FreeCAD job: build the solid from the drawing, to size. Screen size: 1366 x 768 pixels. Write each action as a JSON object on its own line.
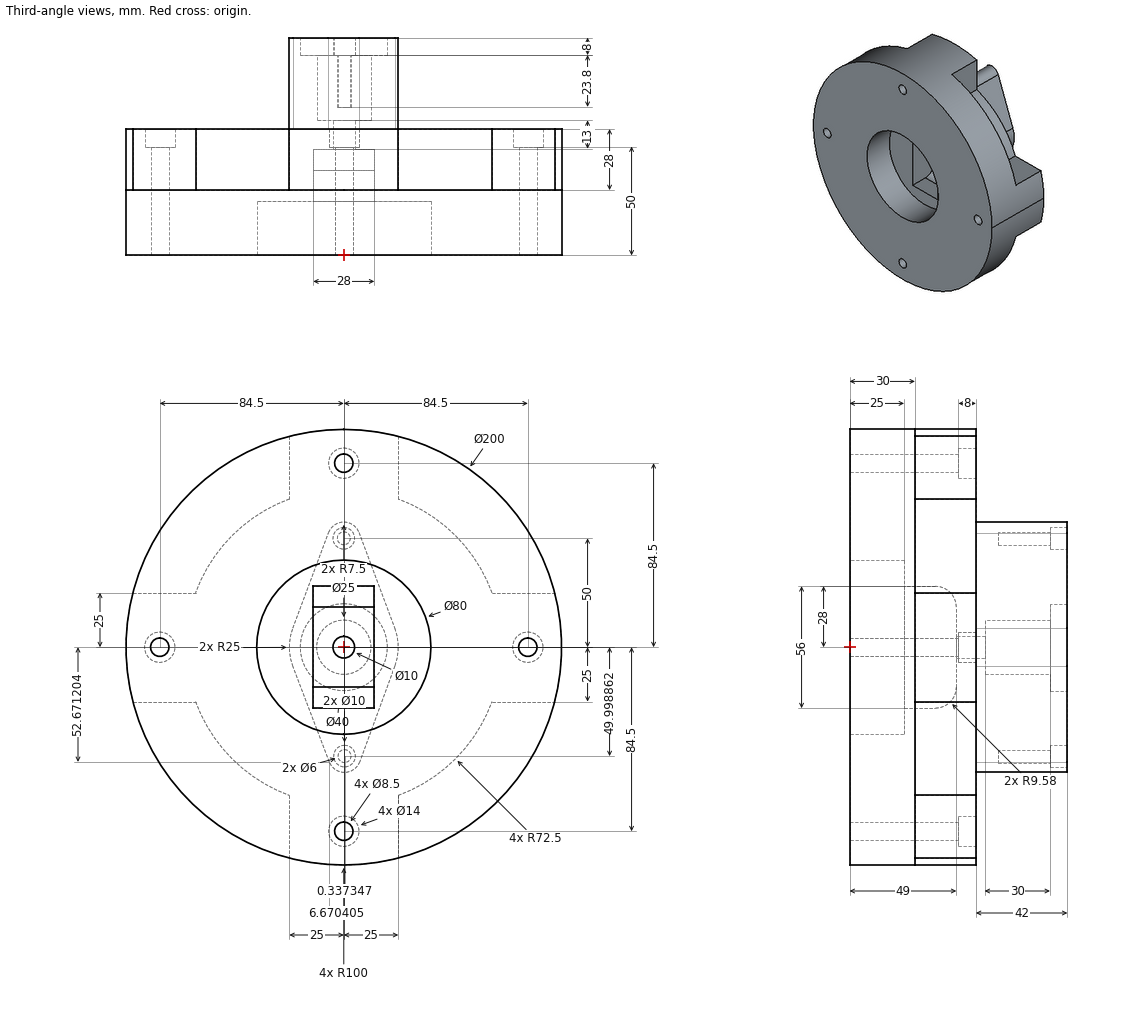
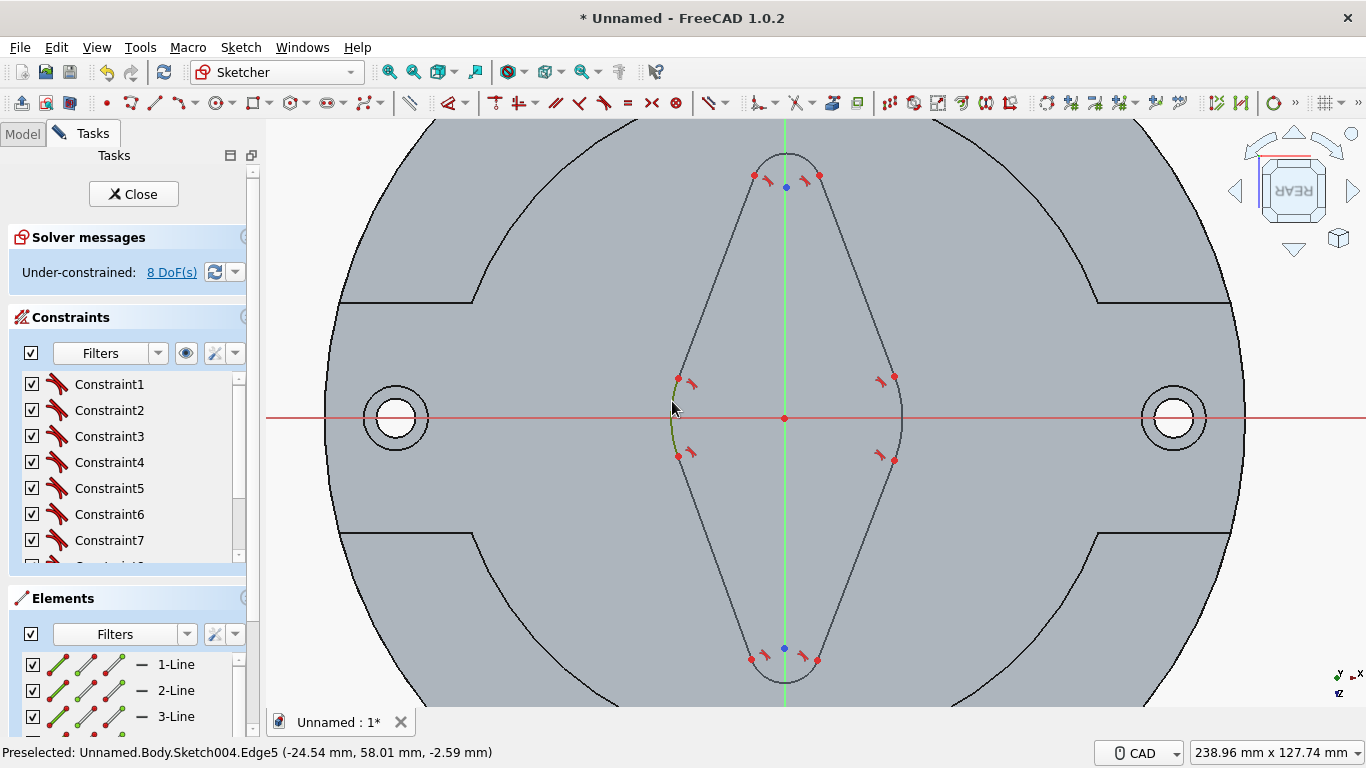
{"action": "left_click", "coordinate": [901, 436]}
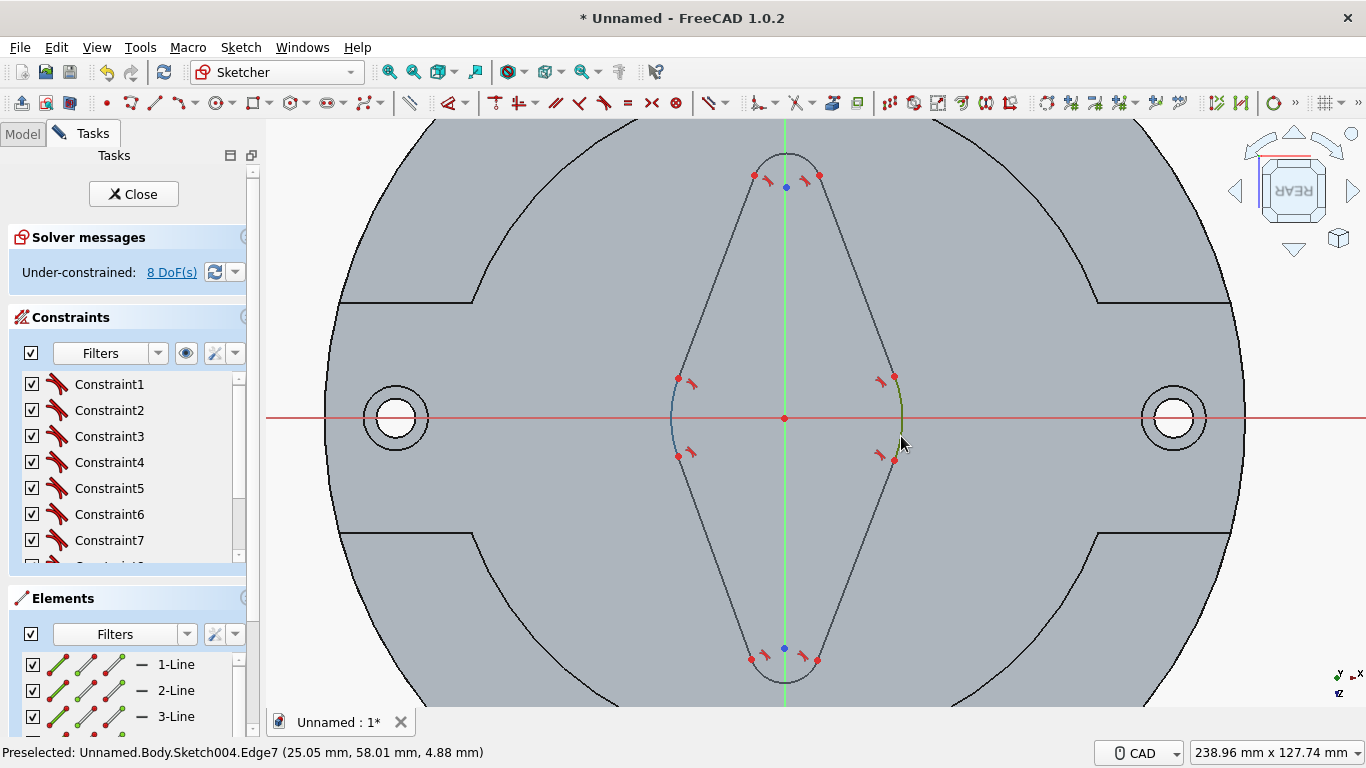
{"action": "key", "text": "e"}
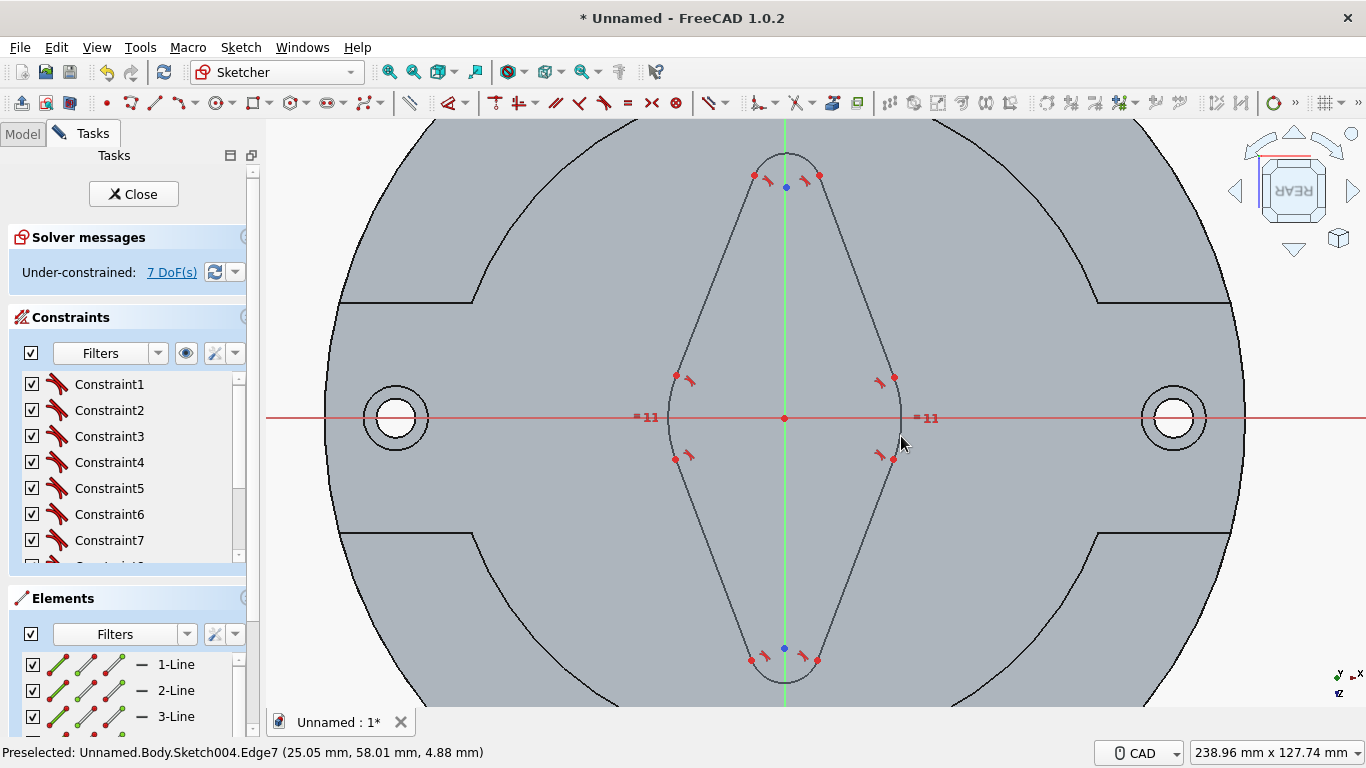
{"action": "left_click", "coordinate": [761, 674]}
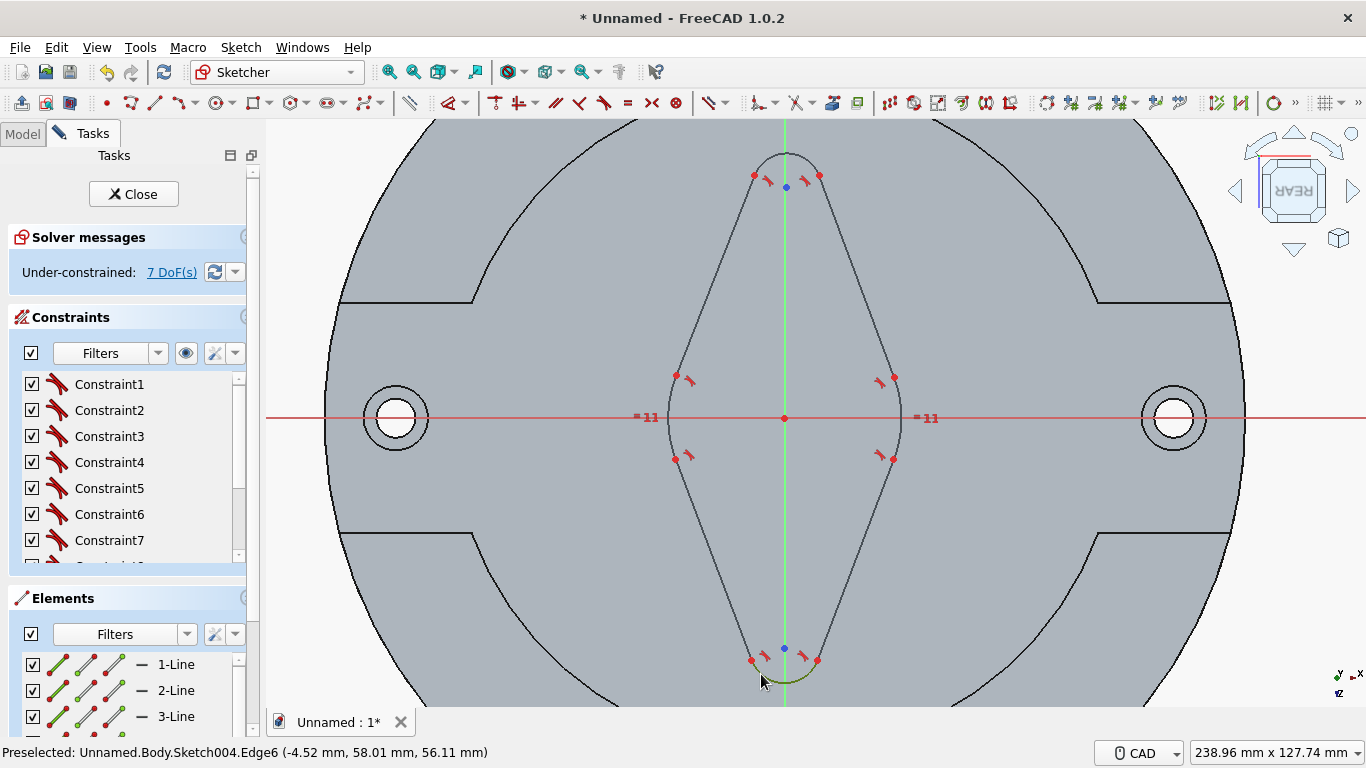
{"action": "left_click", "coordinate": [803, 157]}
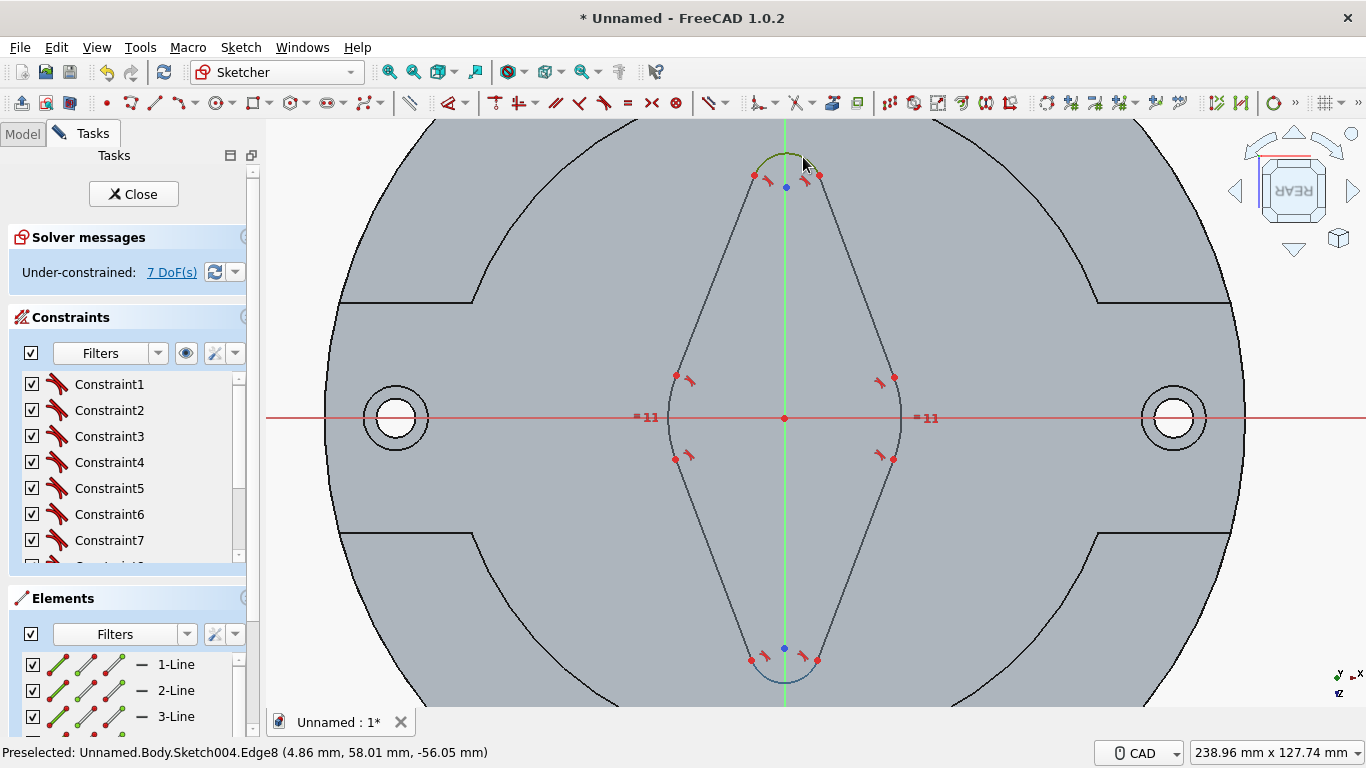
{"action": "key", "text": "e"}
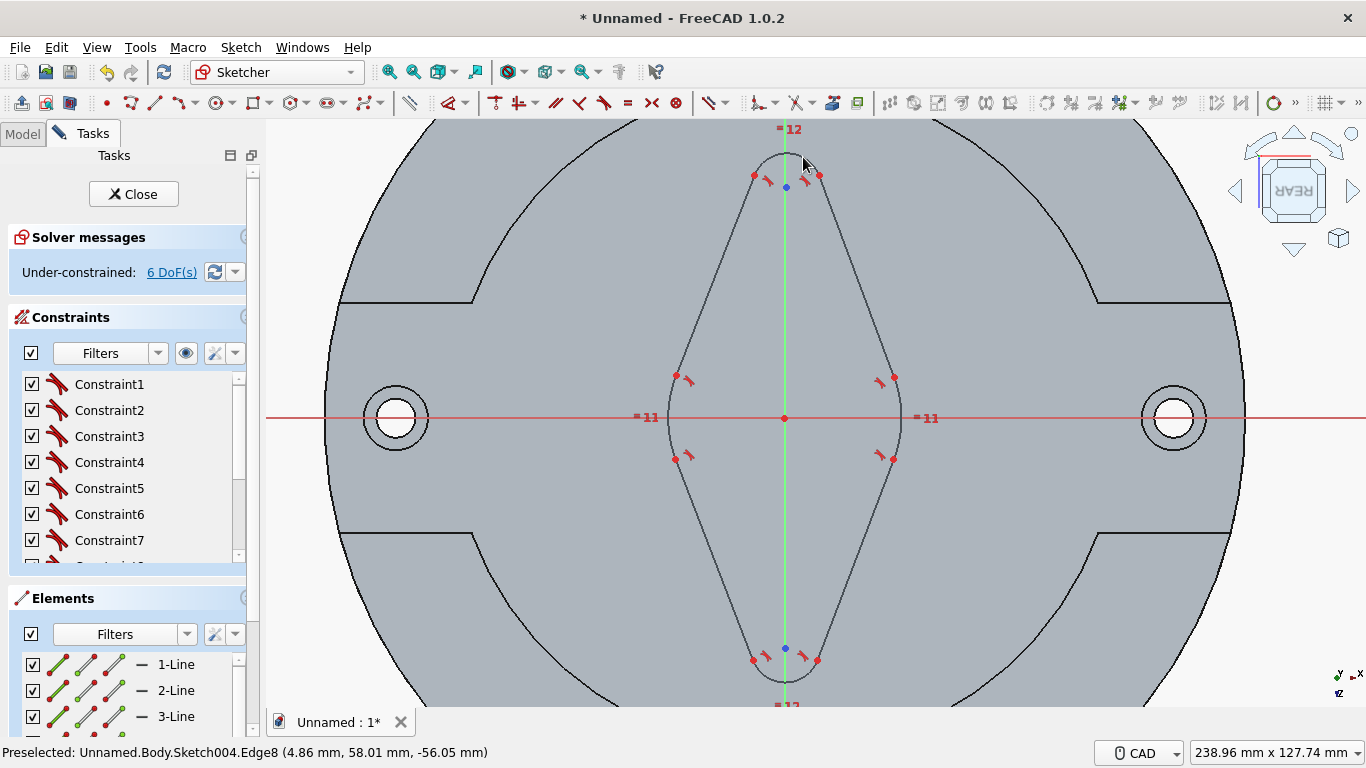
{"action": "left_click", "coordinate": [785, 648]}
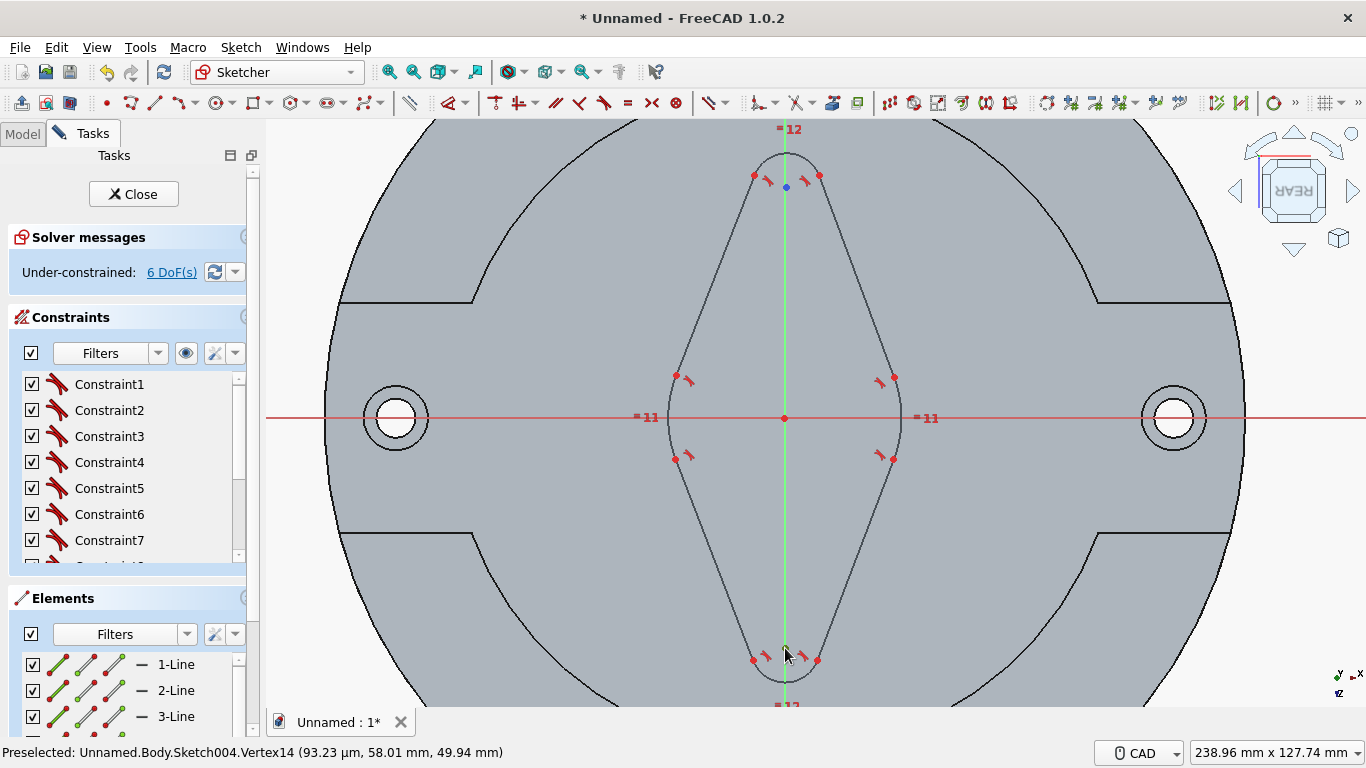
{"action": "left_click", "coordinate": [785, 641]}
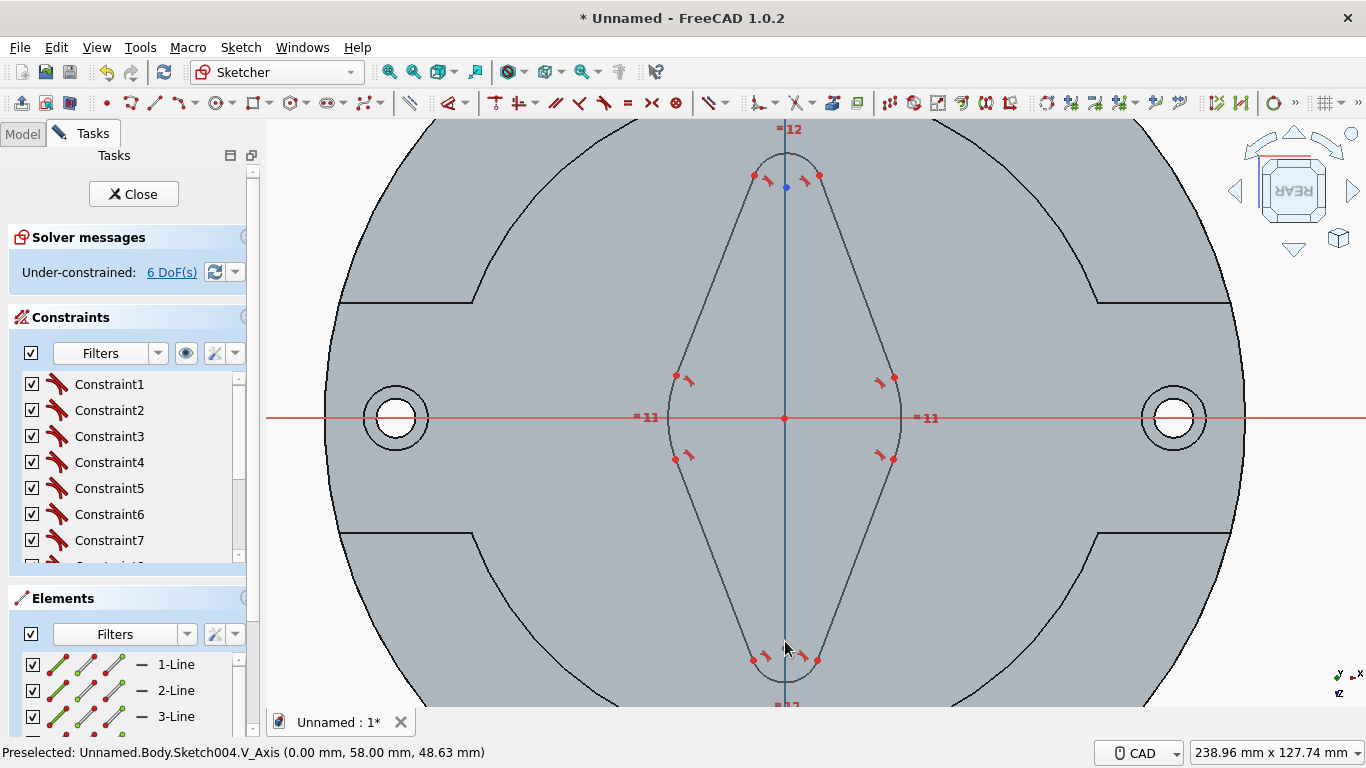
{"action": "left_click", "coordinate": [496, 104]}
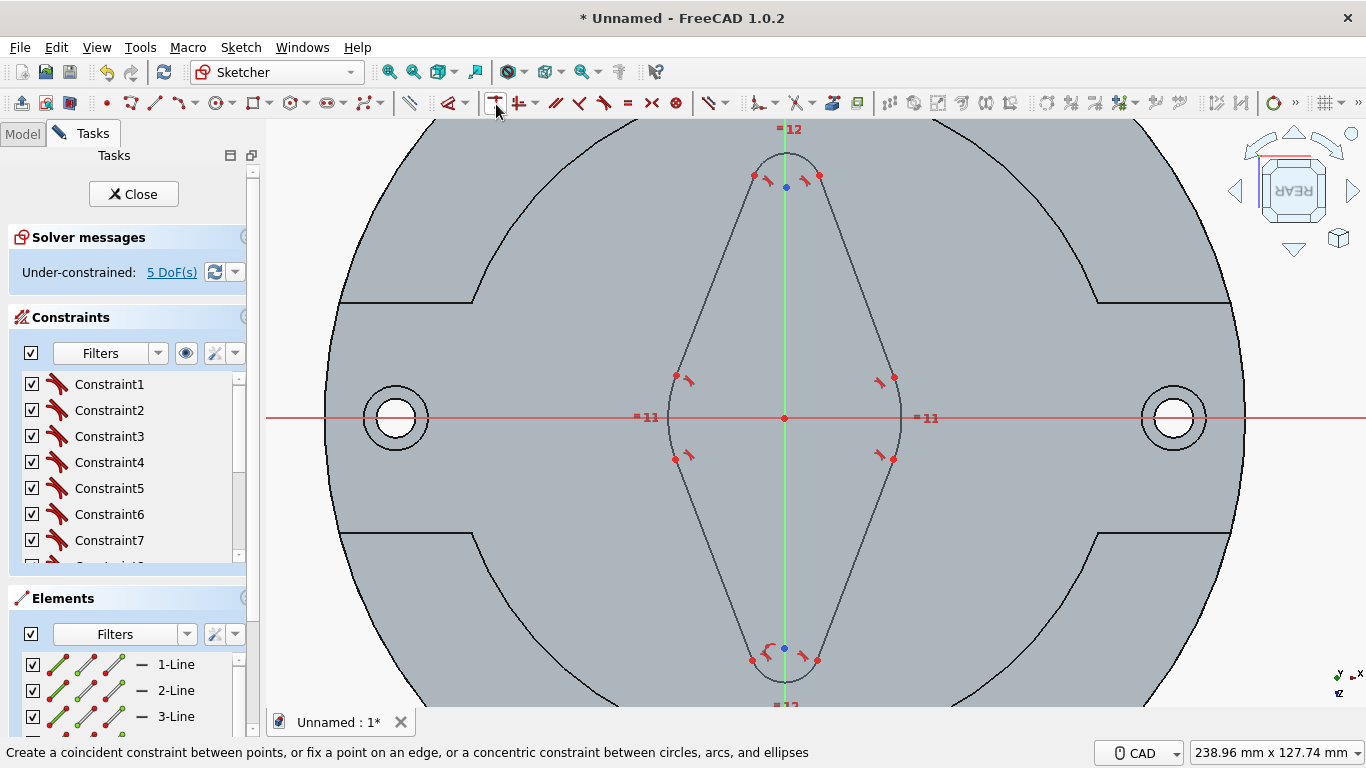
{"action": "key", "text": "d"}